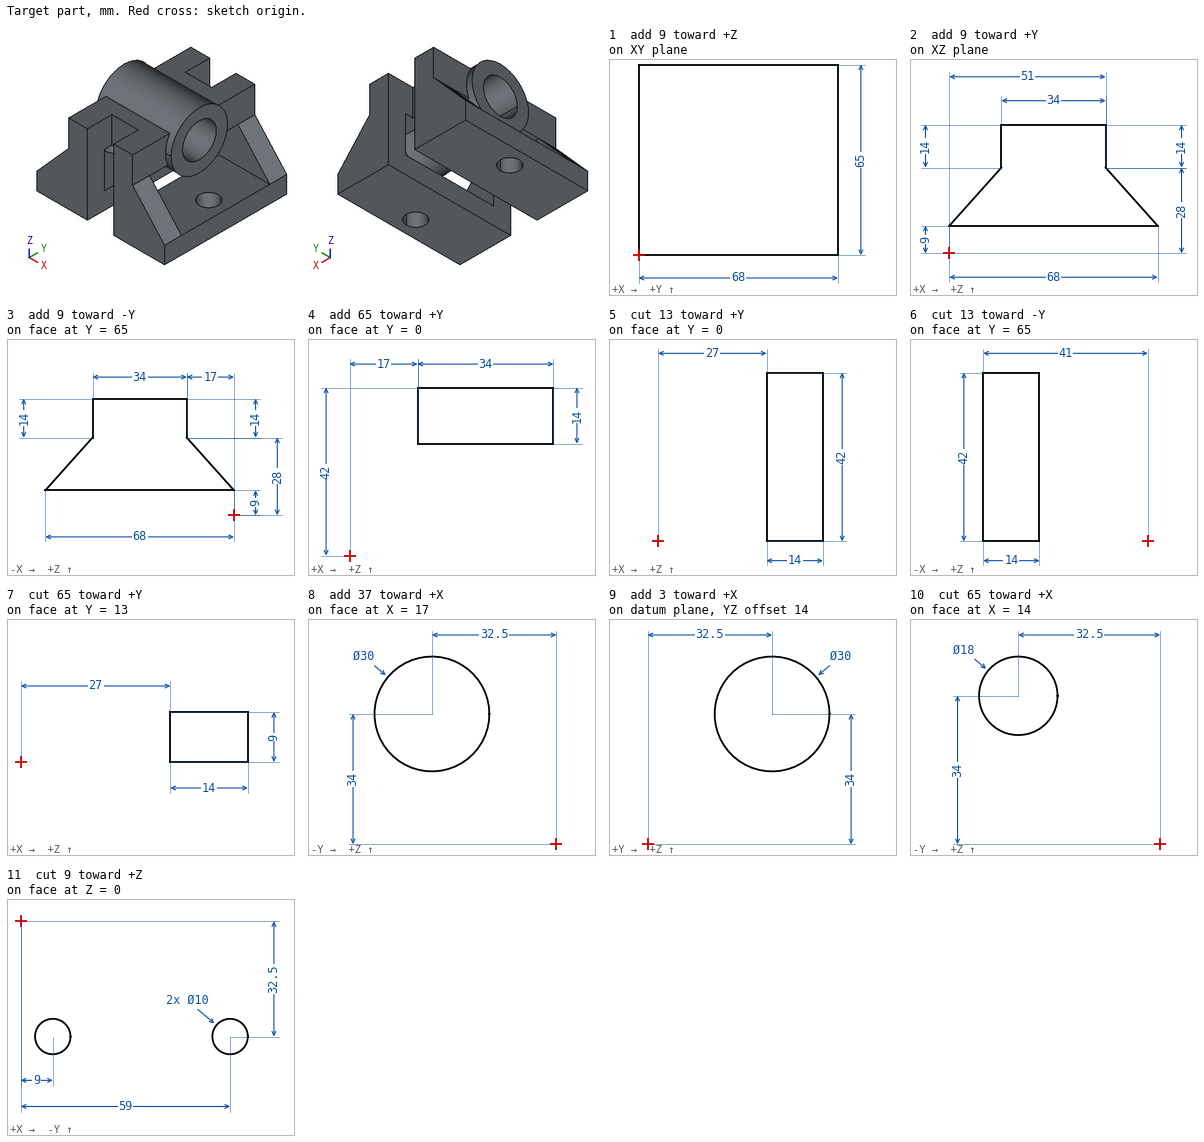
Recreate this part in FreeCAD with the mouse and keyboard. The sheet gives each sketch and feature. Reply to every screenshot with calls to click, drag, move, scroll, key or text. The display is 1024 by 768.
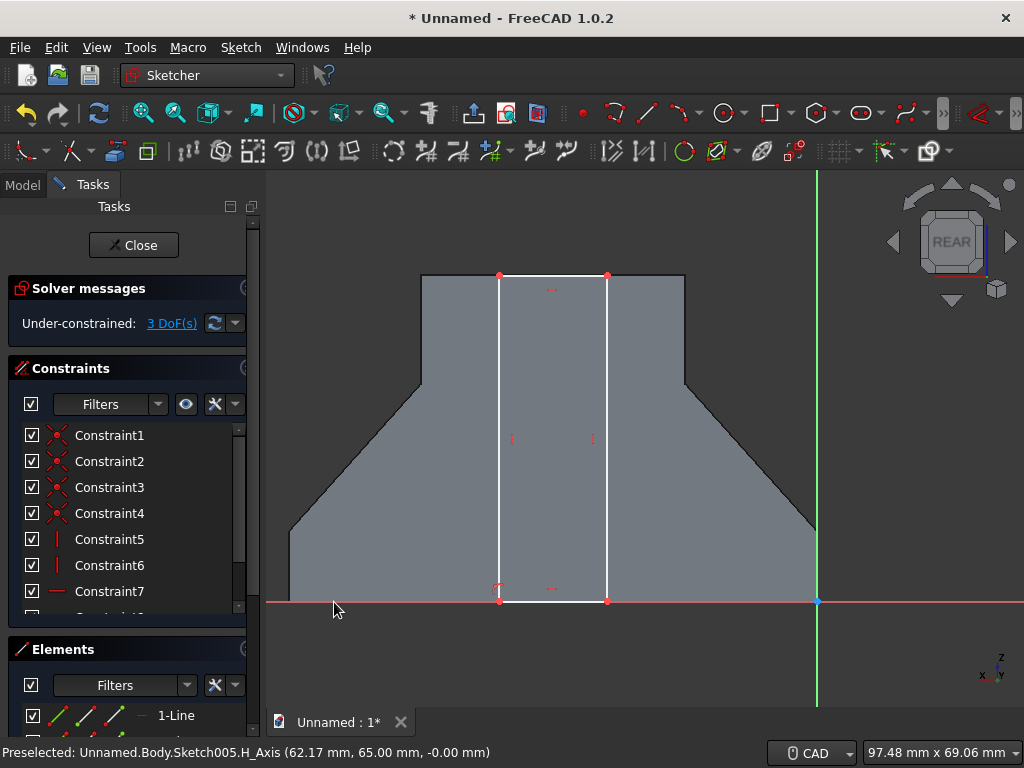
click(978, 114)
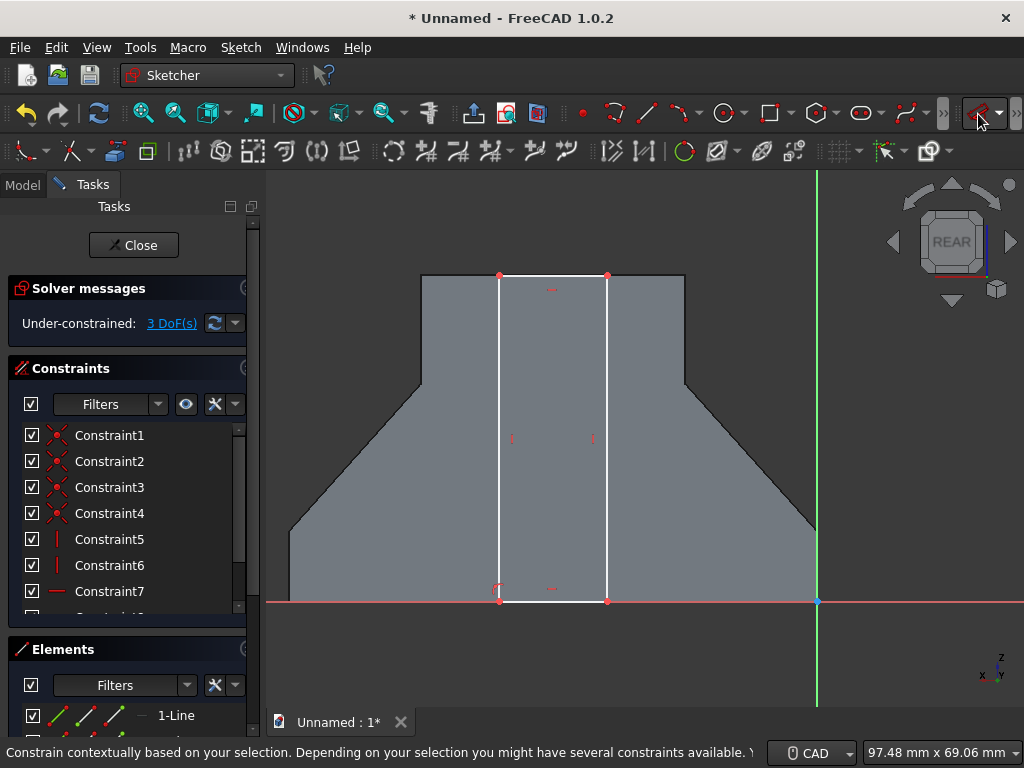
click(499, 374)
click(465, 439)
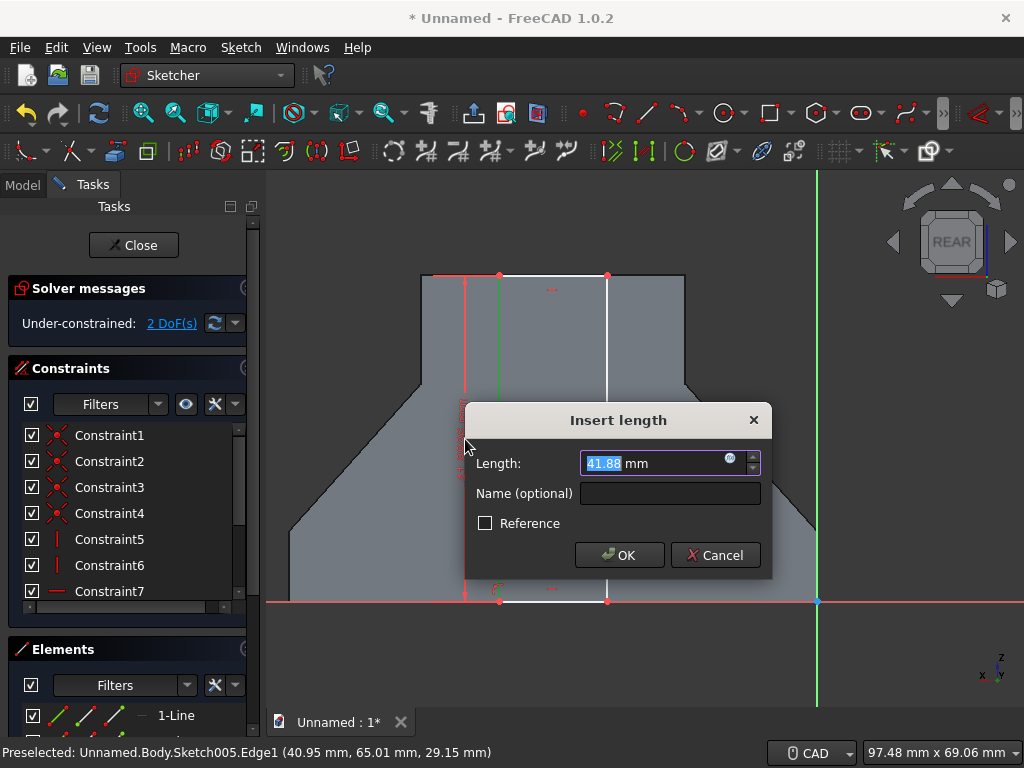
text(42)
key(Return)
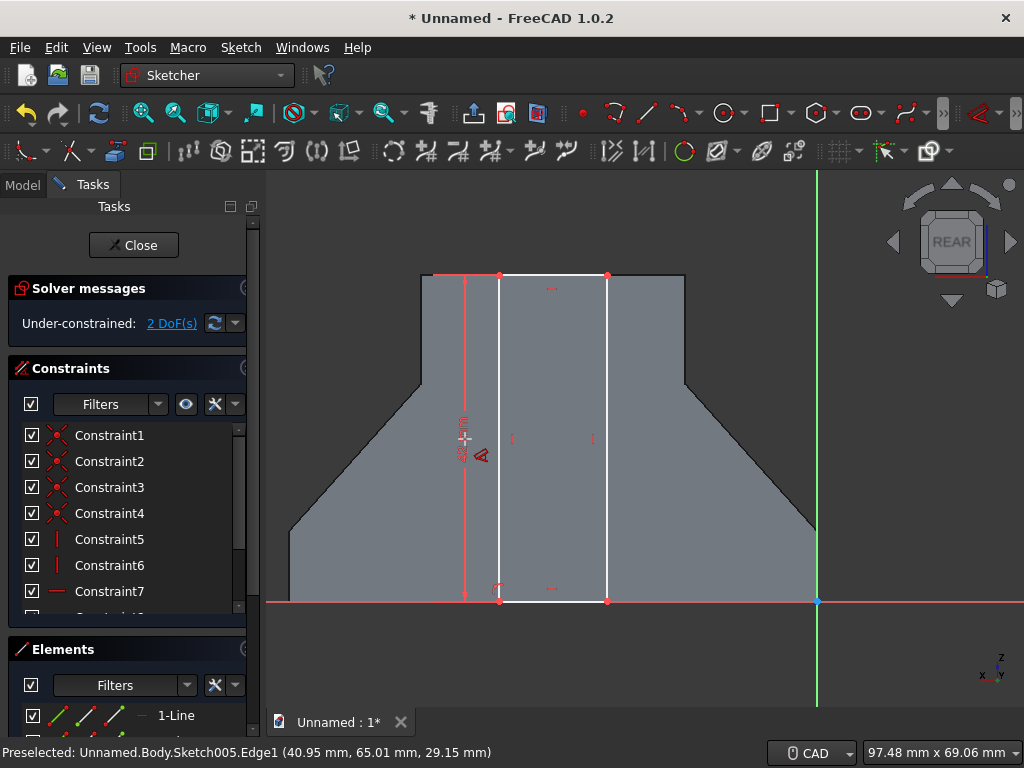
click(531, 602)
click(553, 636)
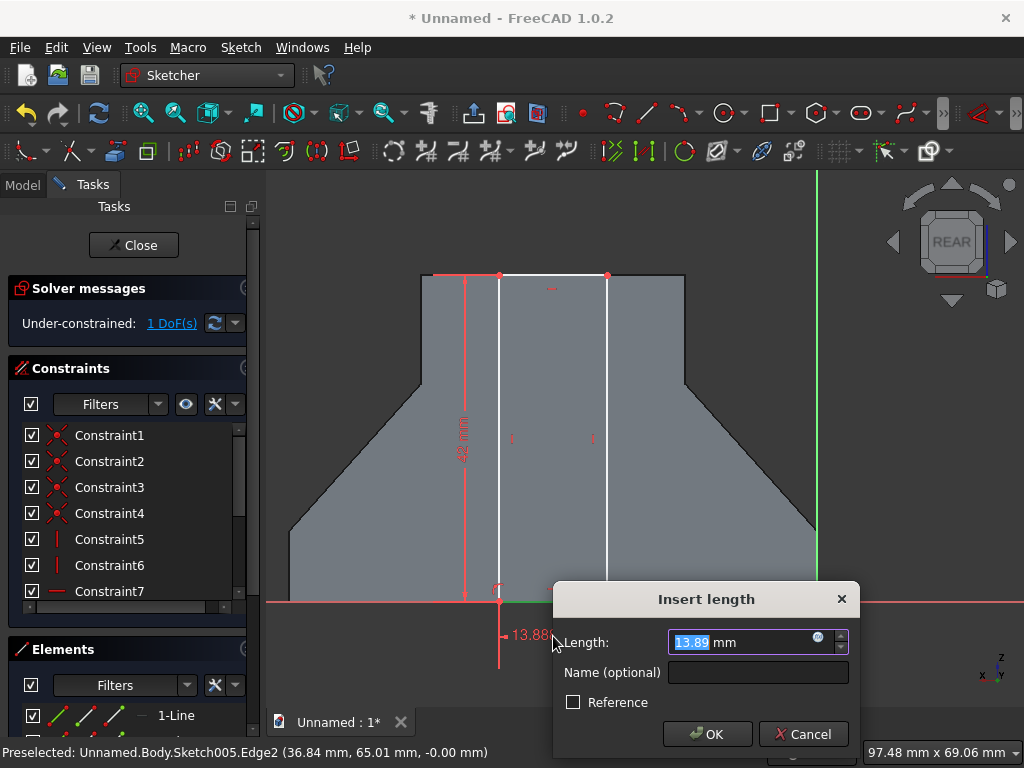
text(14)
key(Return)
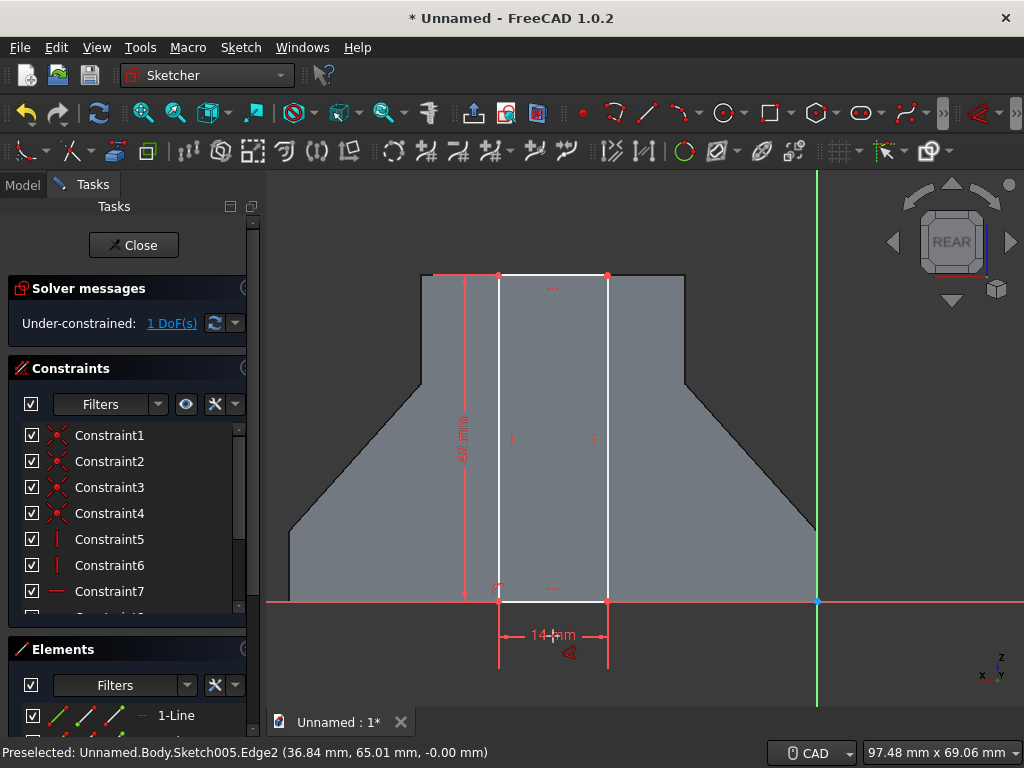
click(499, 275)
click(658, 636)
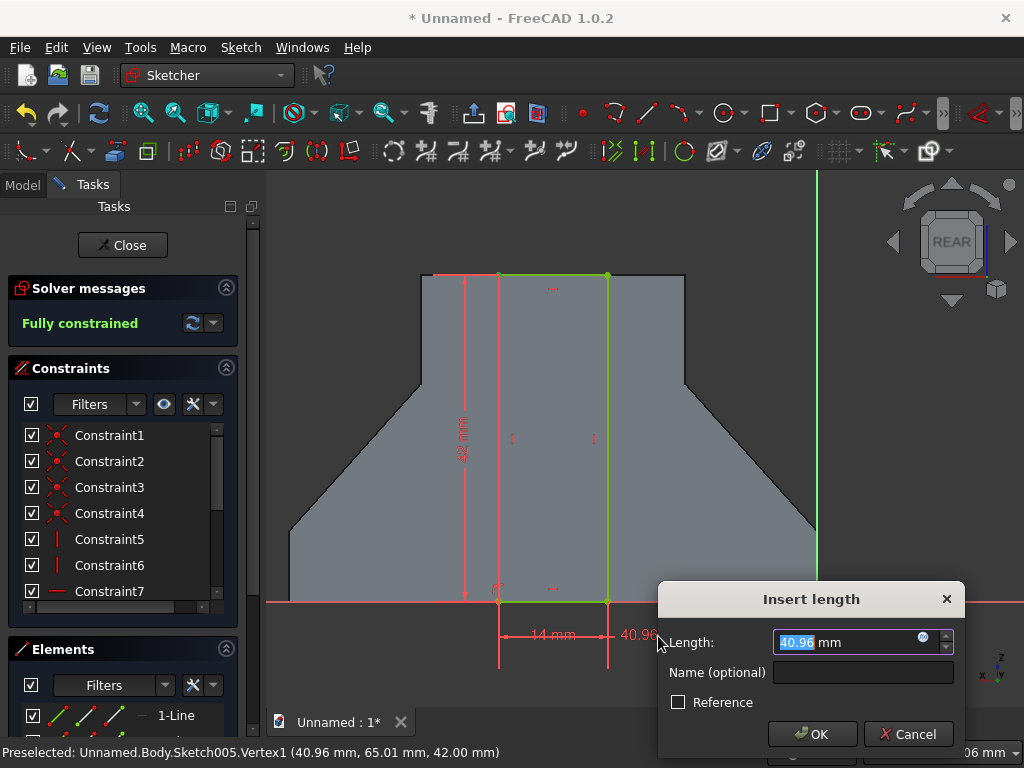
text(41)
key(Return)
key(Escape)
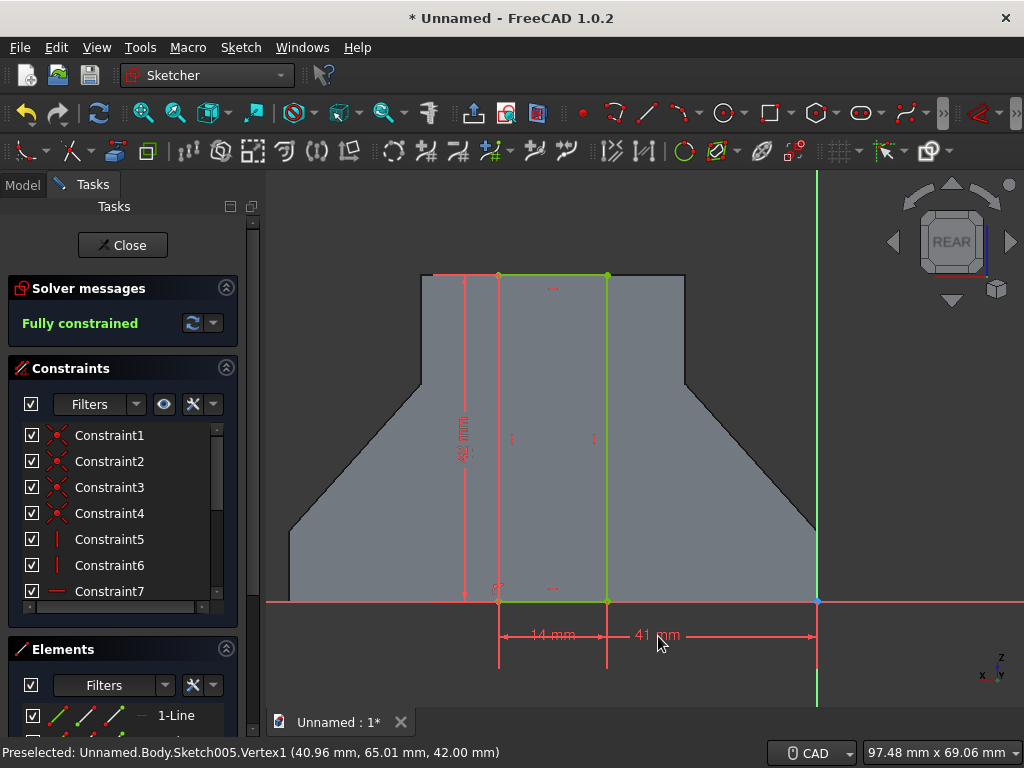
click(123, 245)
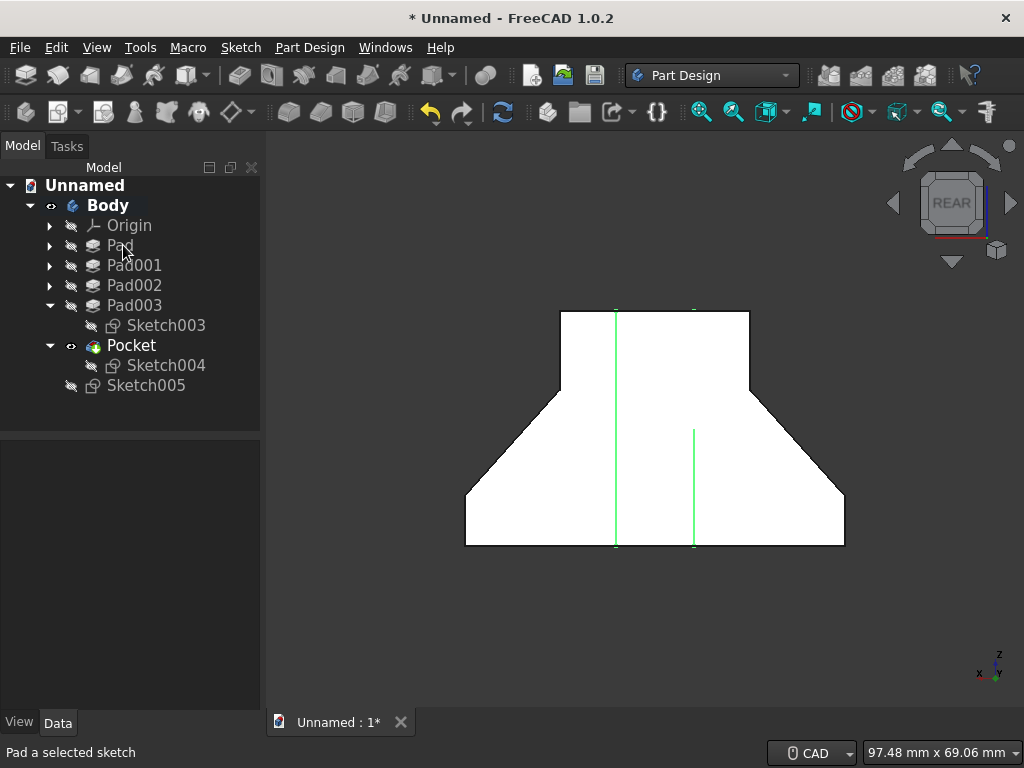
click(240, 76)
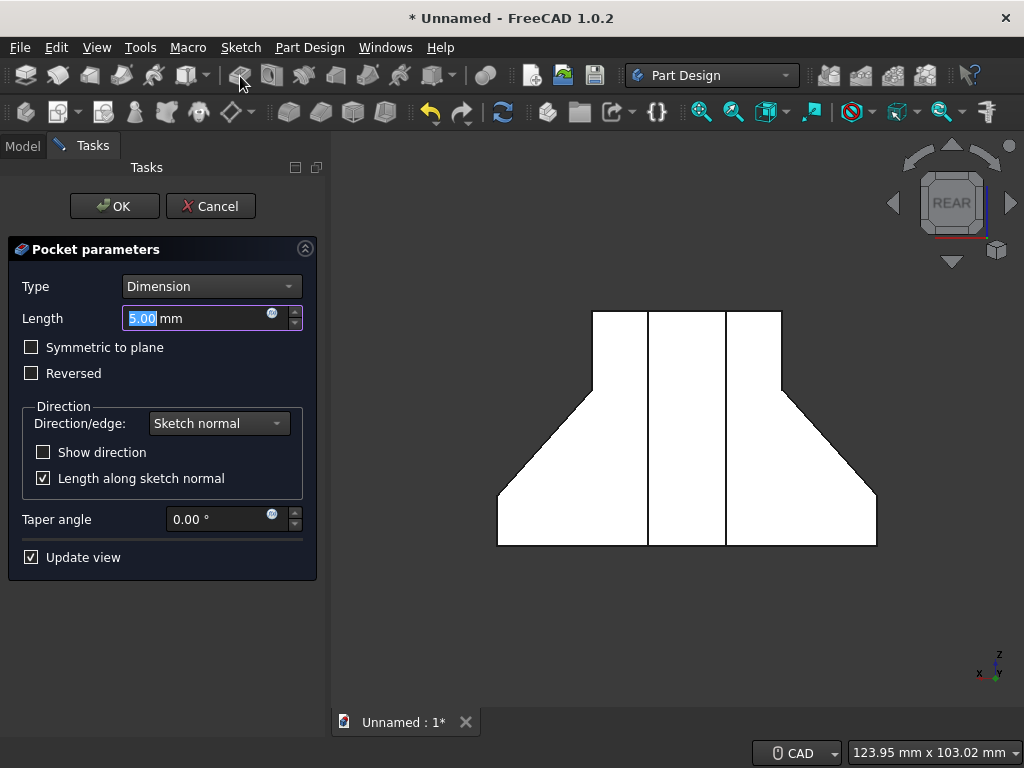
text(13)
key(Tab)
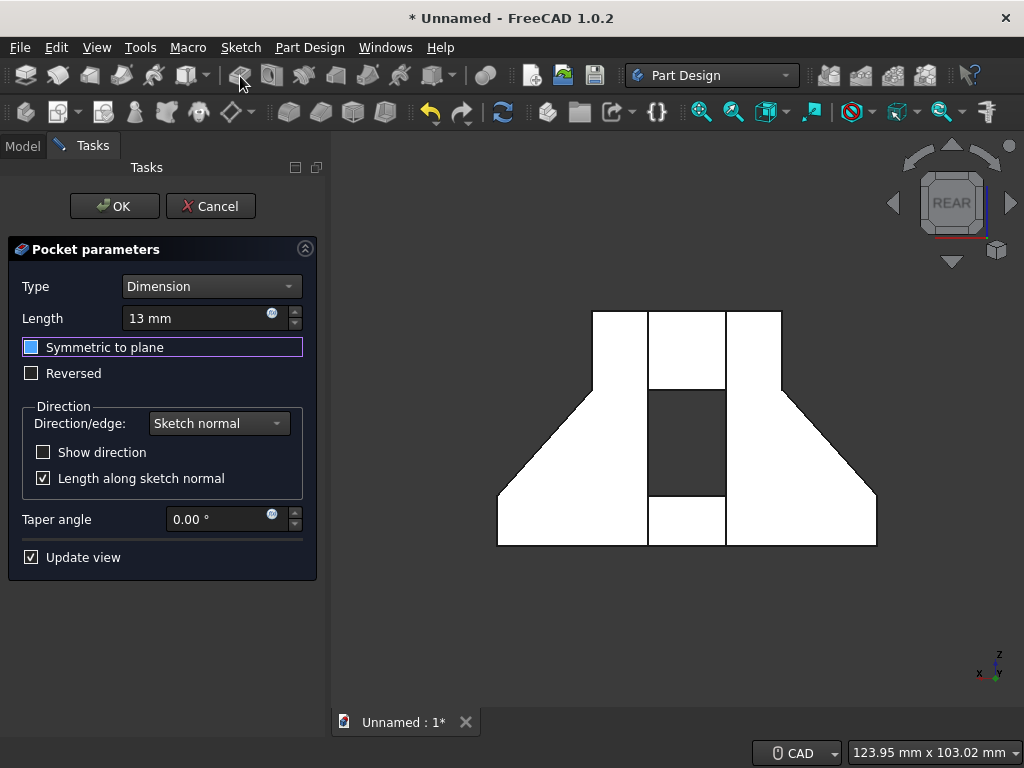
click(115, 206)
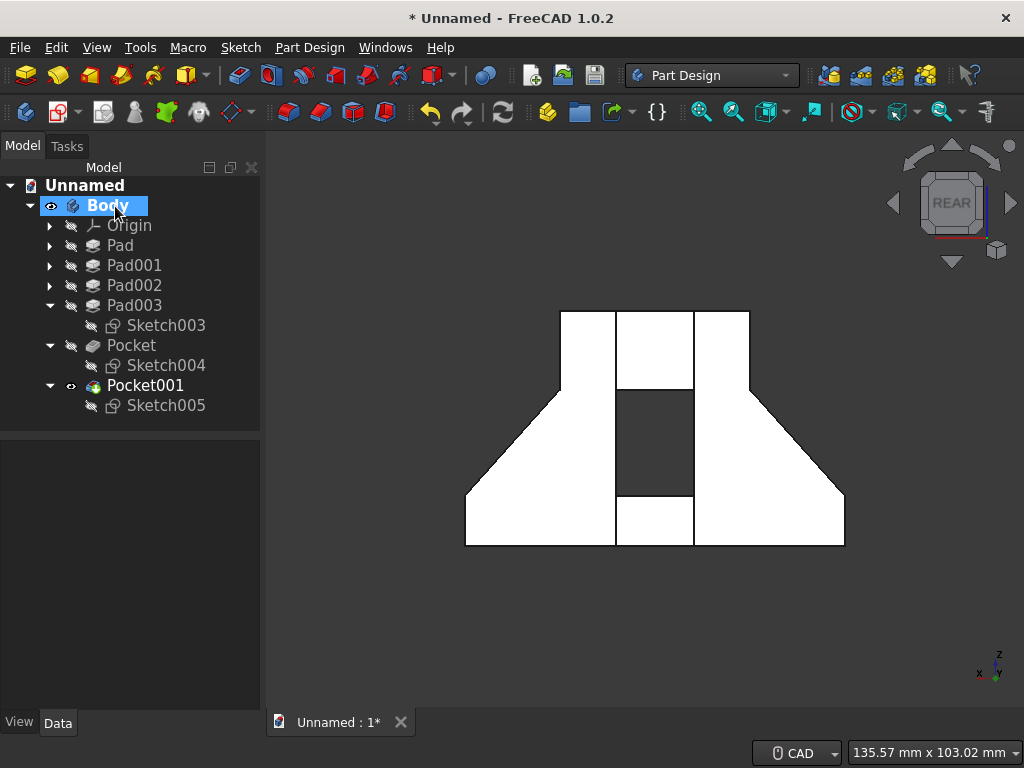
key(0)